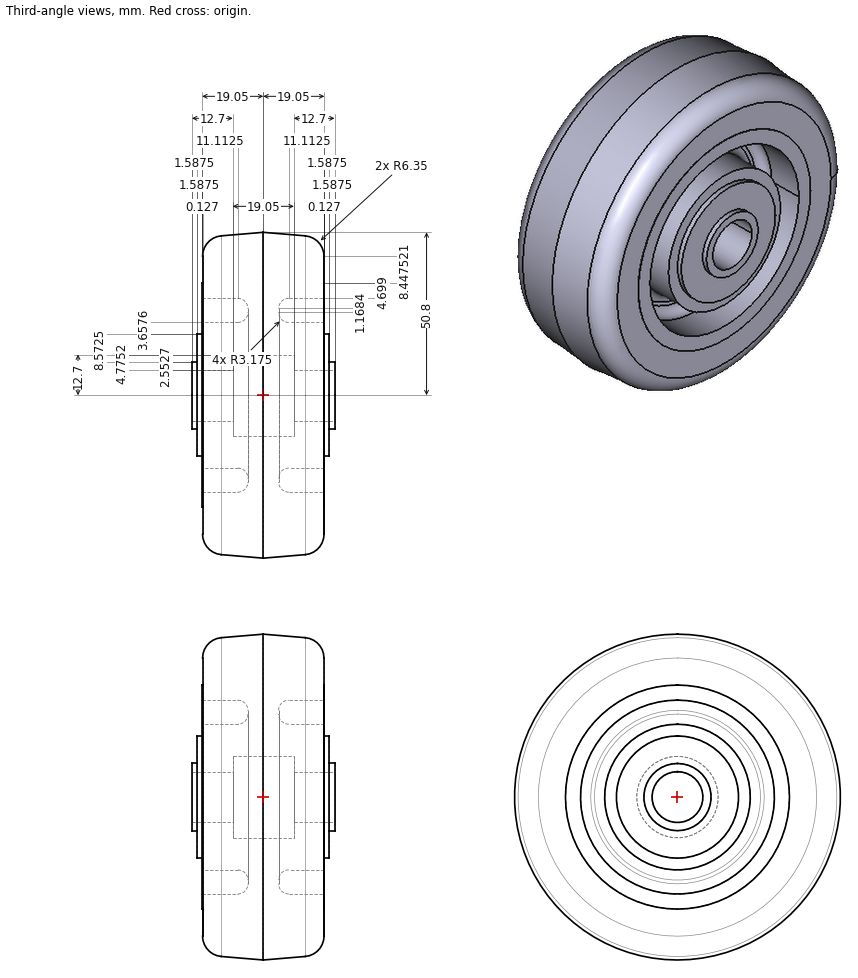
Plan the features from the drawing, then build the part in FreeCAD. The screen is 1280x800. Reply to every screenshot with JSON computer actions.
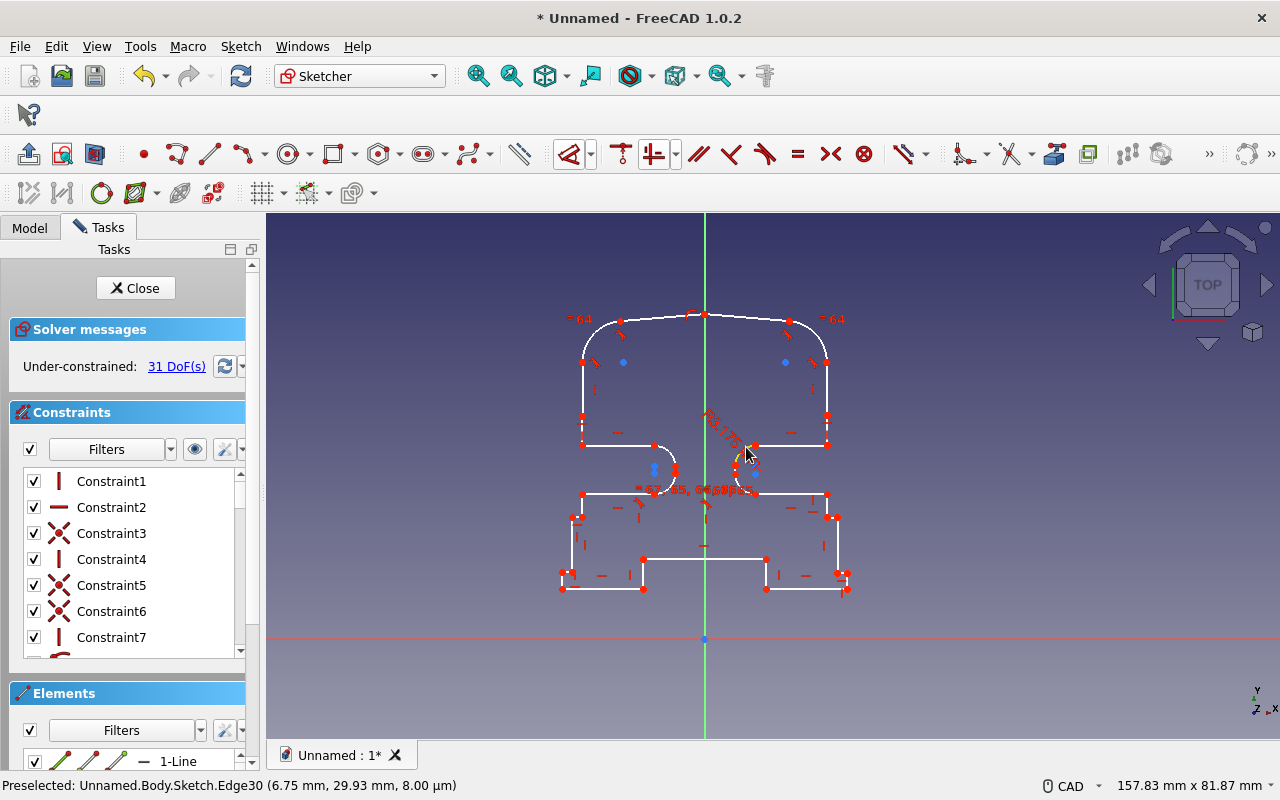
{"action": "left_click", "coordinate": [823, 344]}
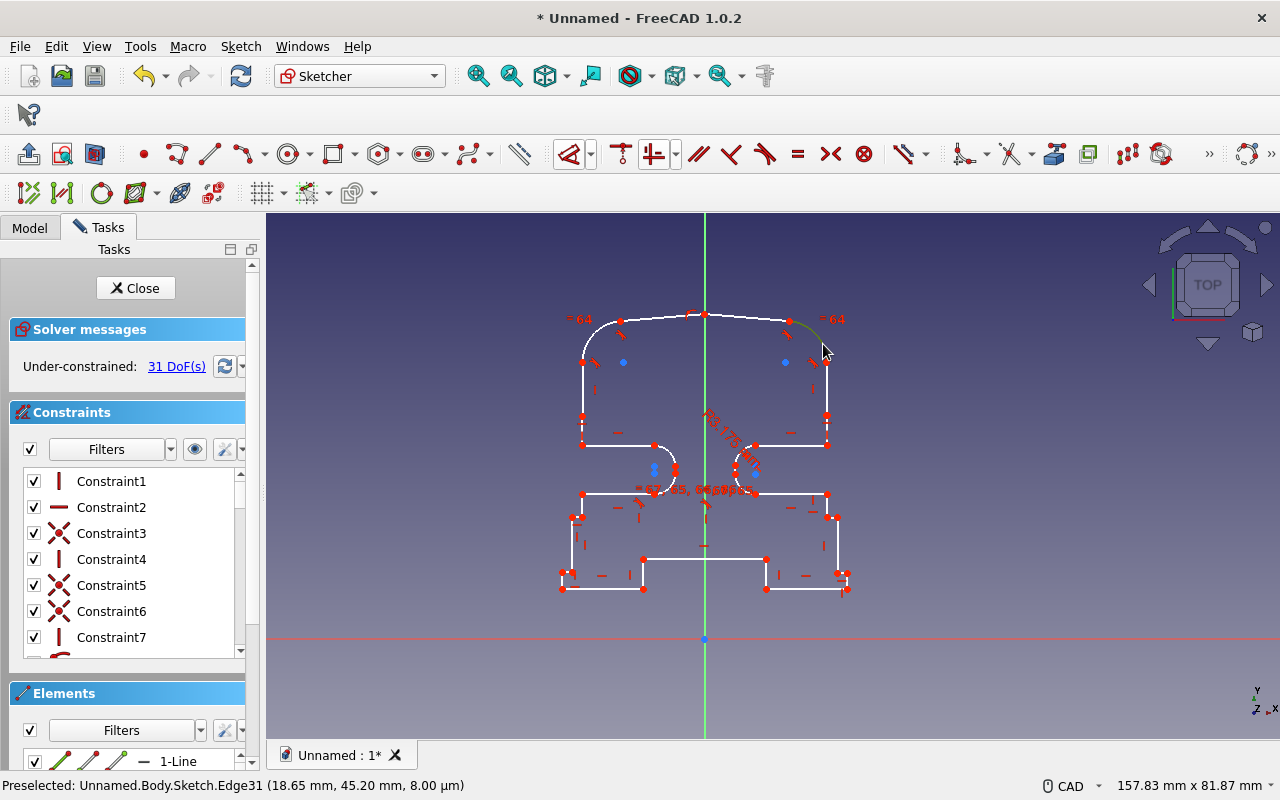
{"action": "left_click", "coordinate": [590, 154]}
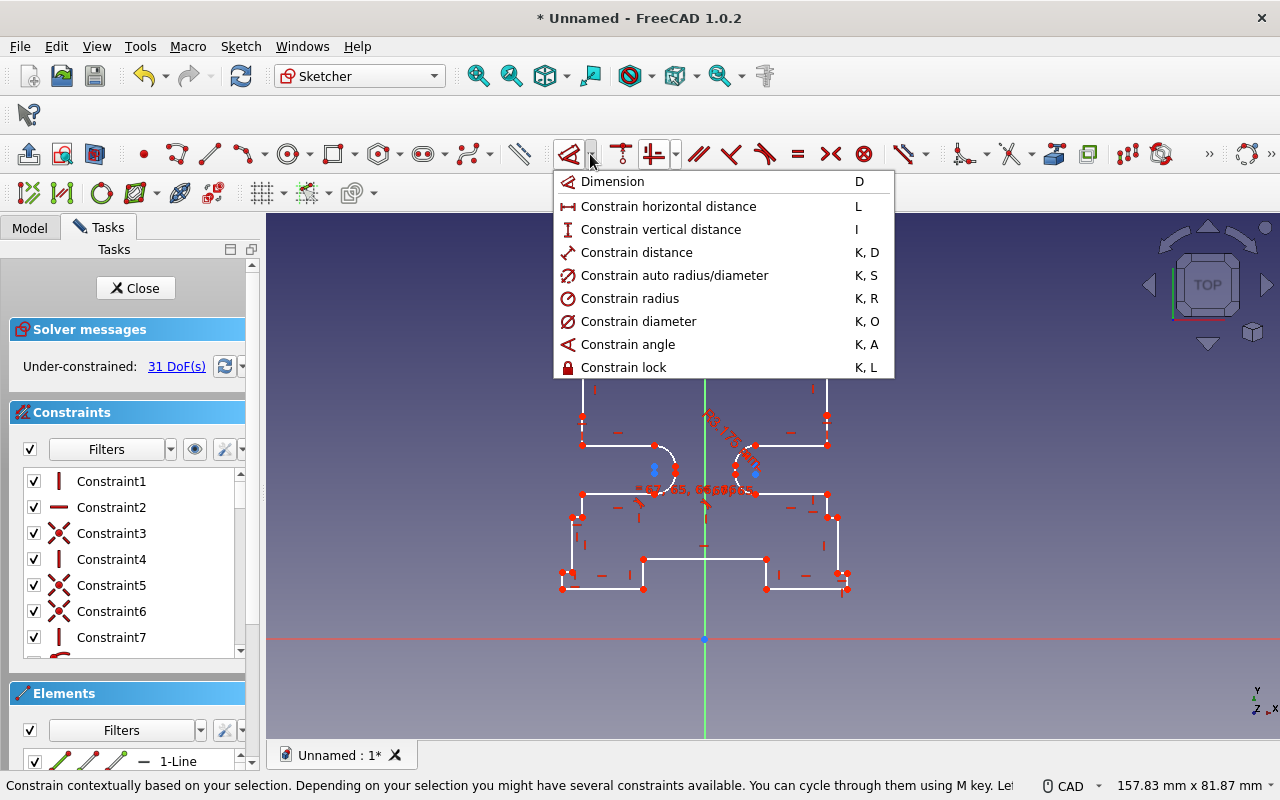
{"action": "left_click", "coordinate": [724, 298]}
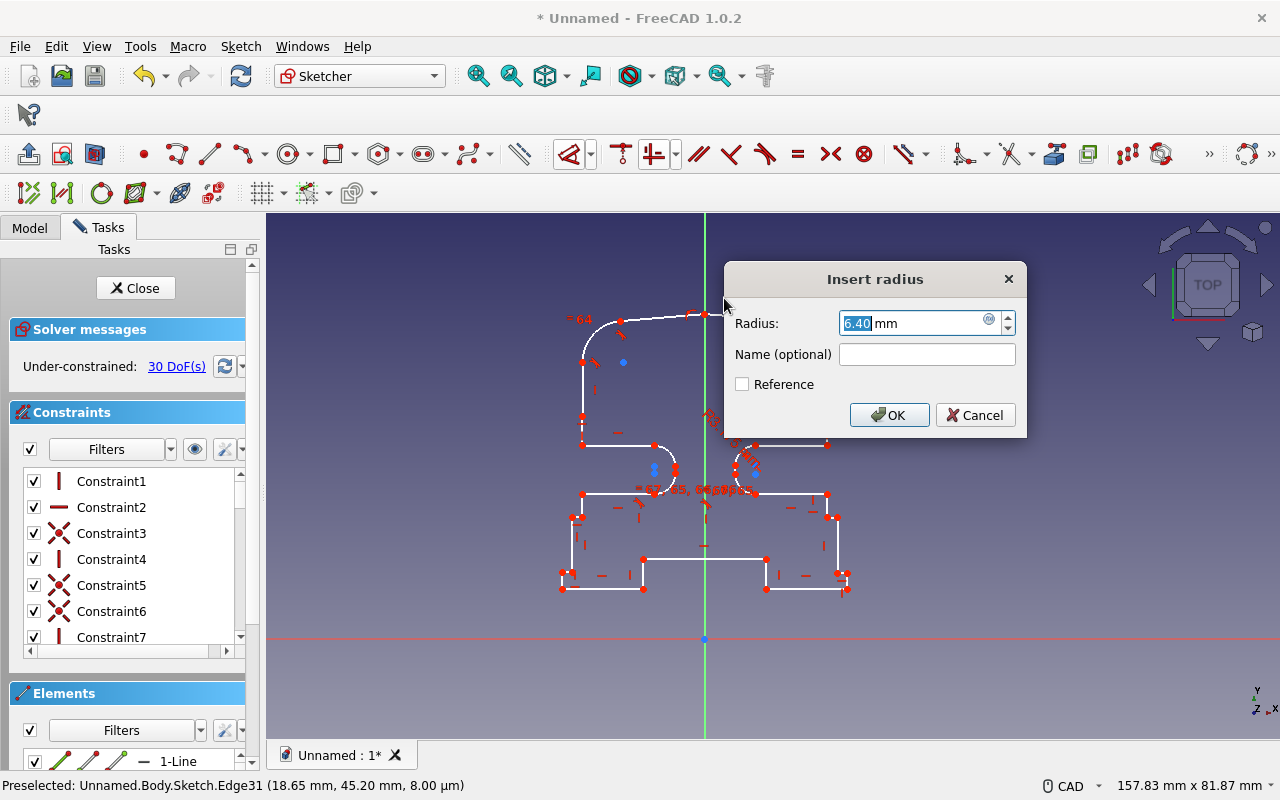
{"action": "type", "text": "6.35"}
{"action": "key", "text": "Return"}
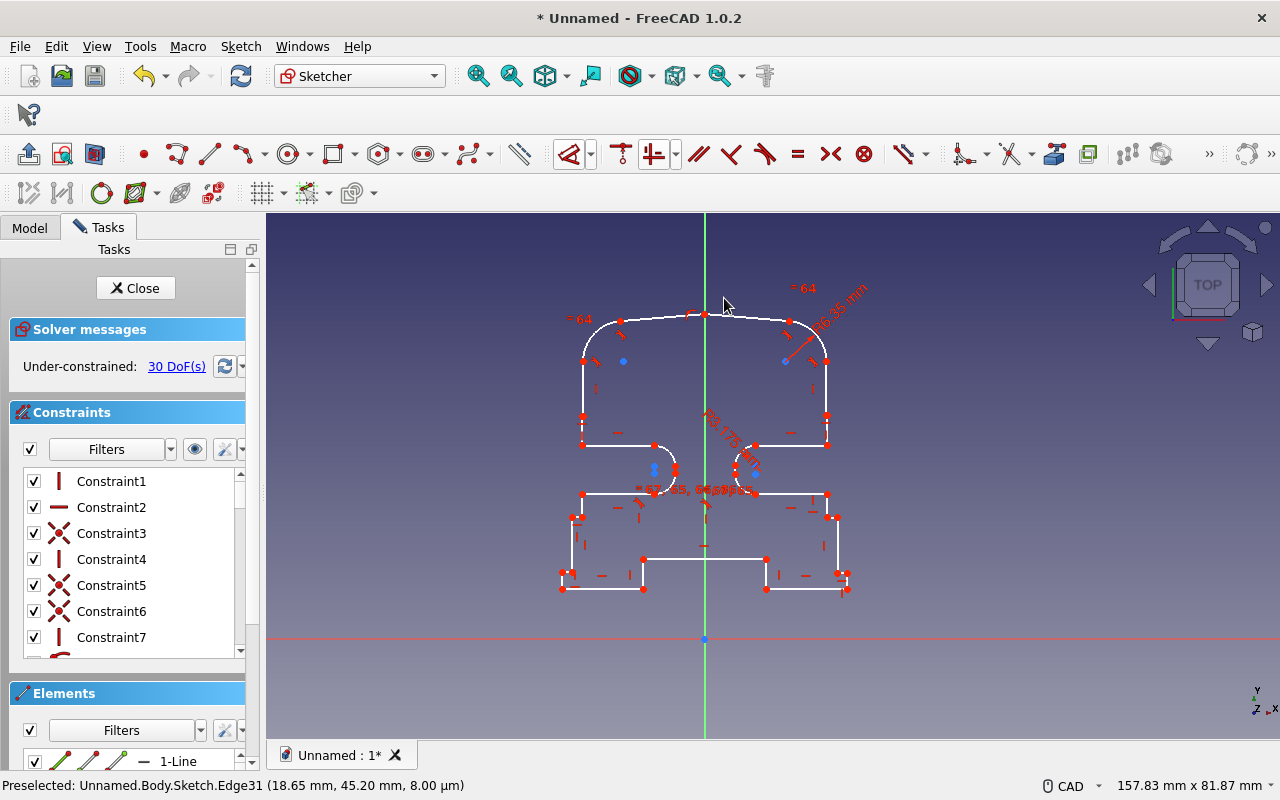
{"action": "left_click", "coordinate": [587, 589]}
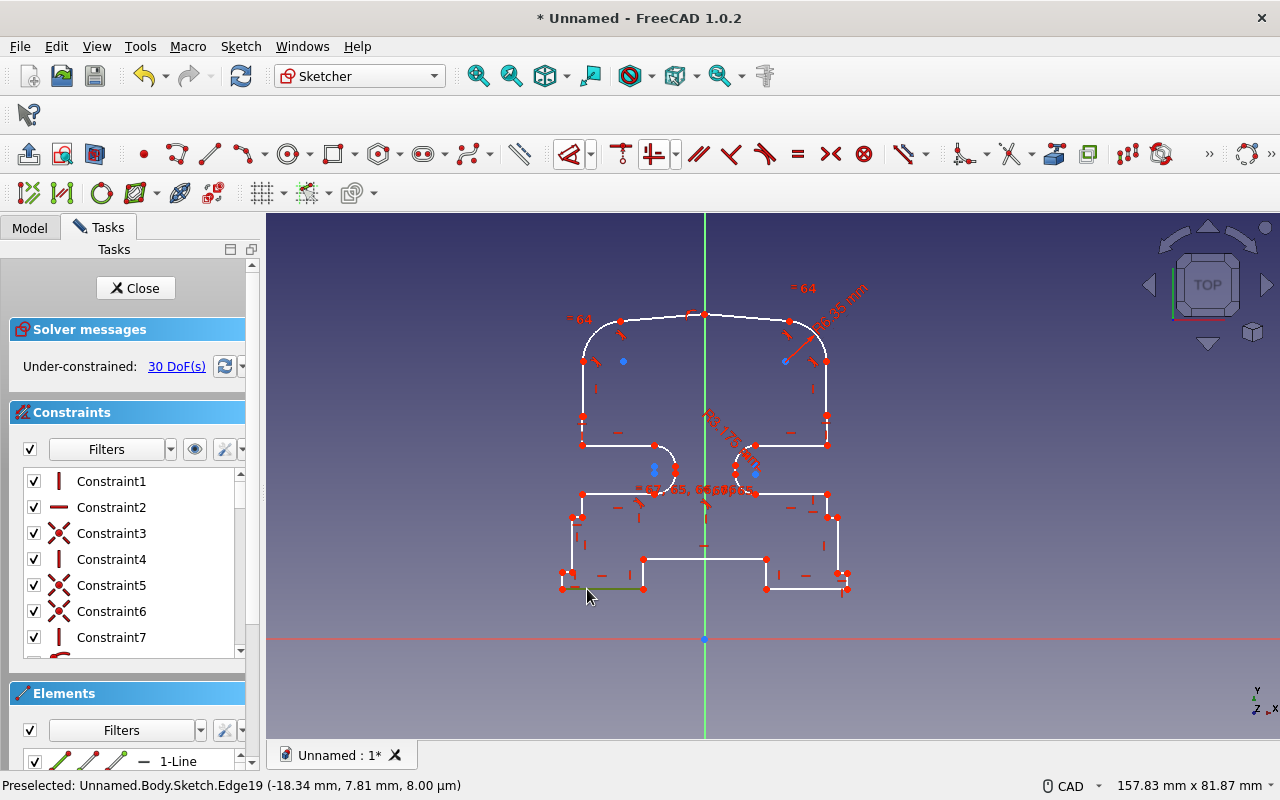
{"action": "left_click", "coordinate": [590, 154]}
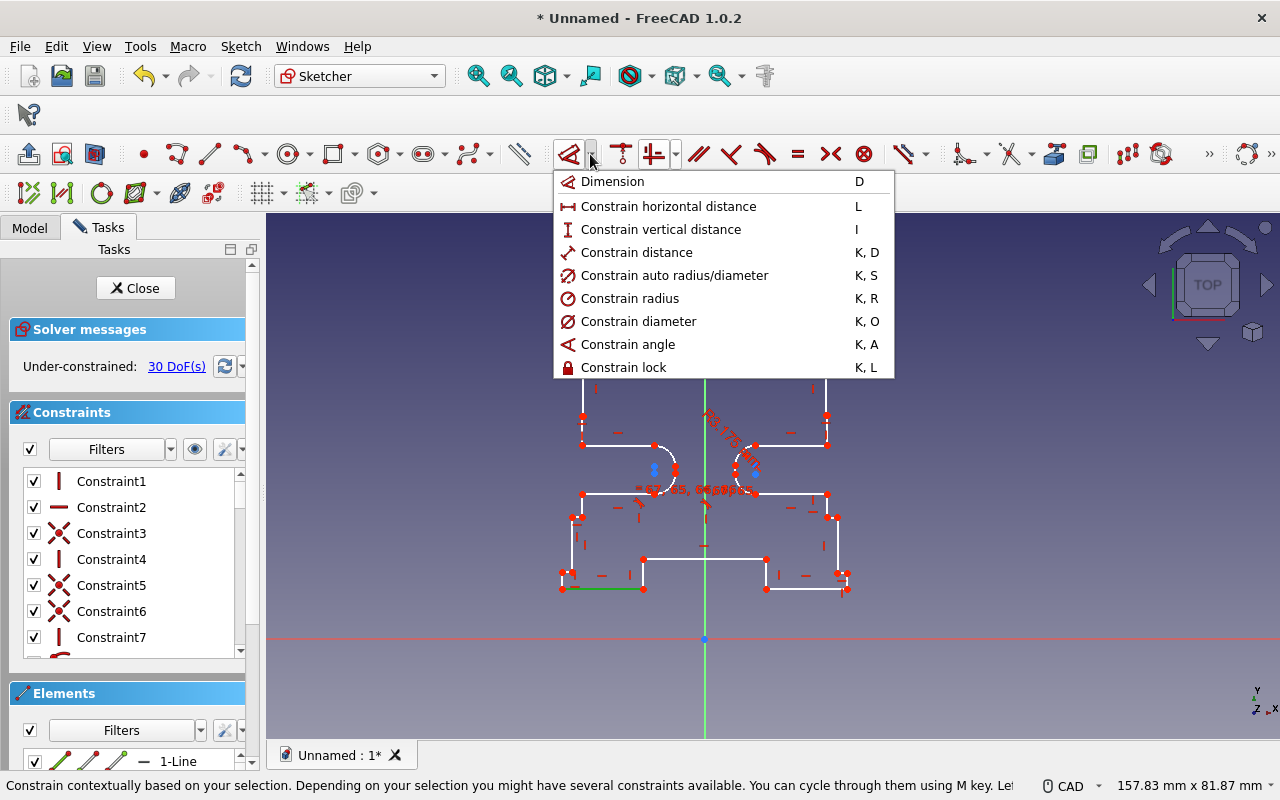
{"action": "left_click", "coordinate": [724, 206]}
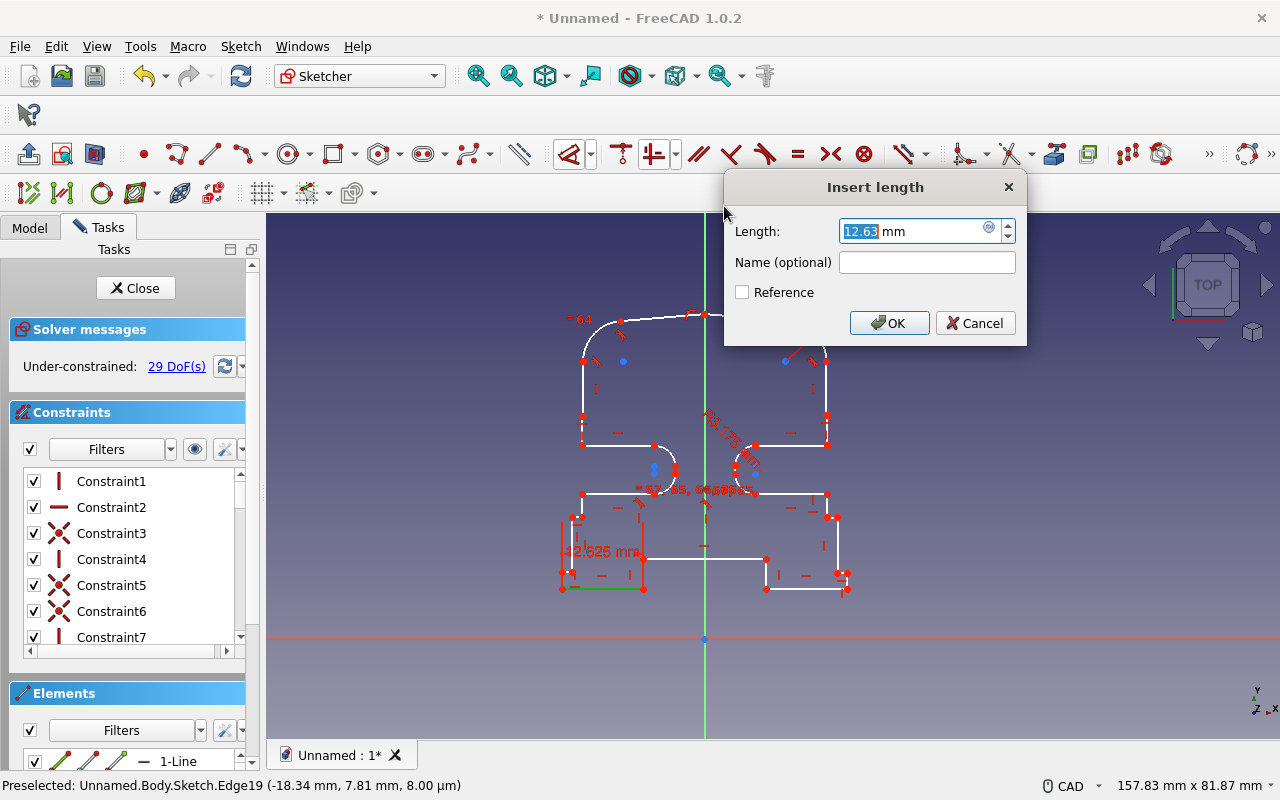
{"action": "type", "text": "12.7"}
{"action": "key", "text": "Return"}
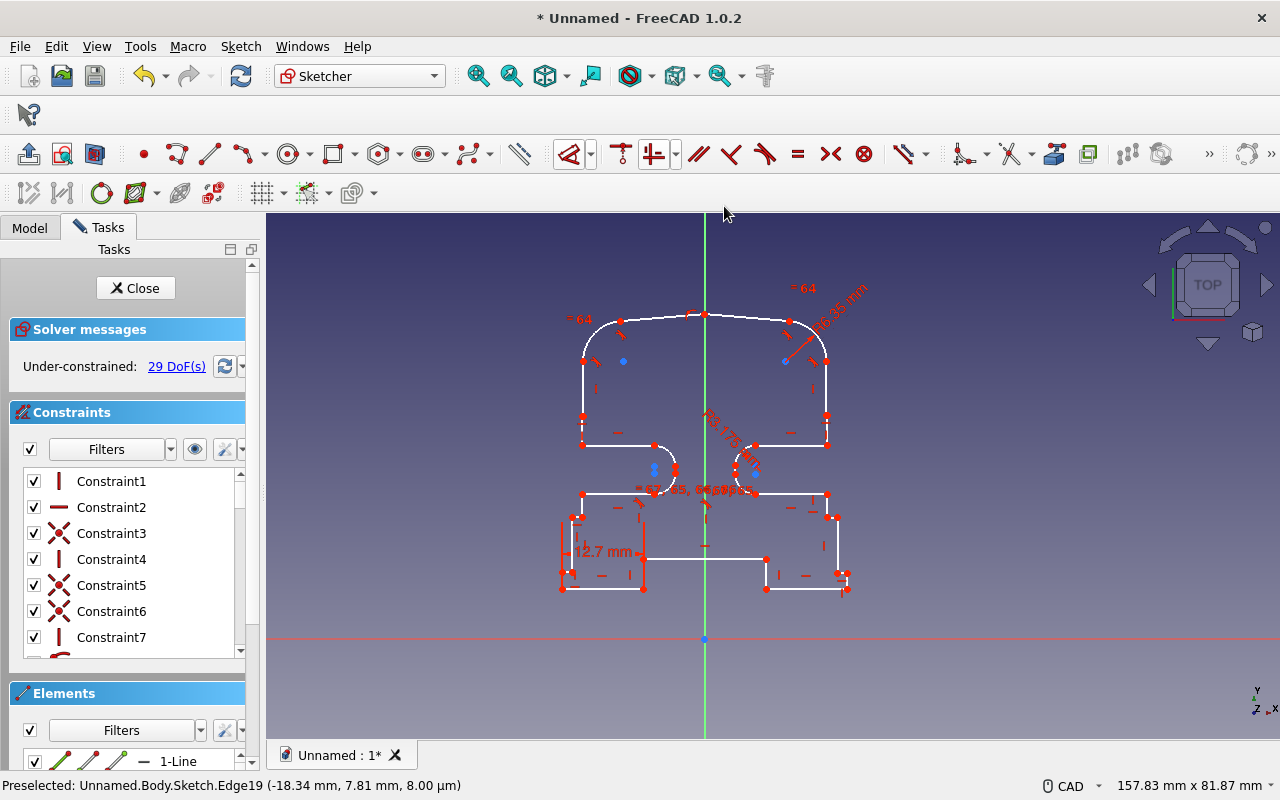
{"action": "left_click", "coordinate": [791, 589]}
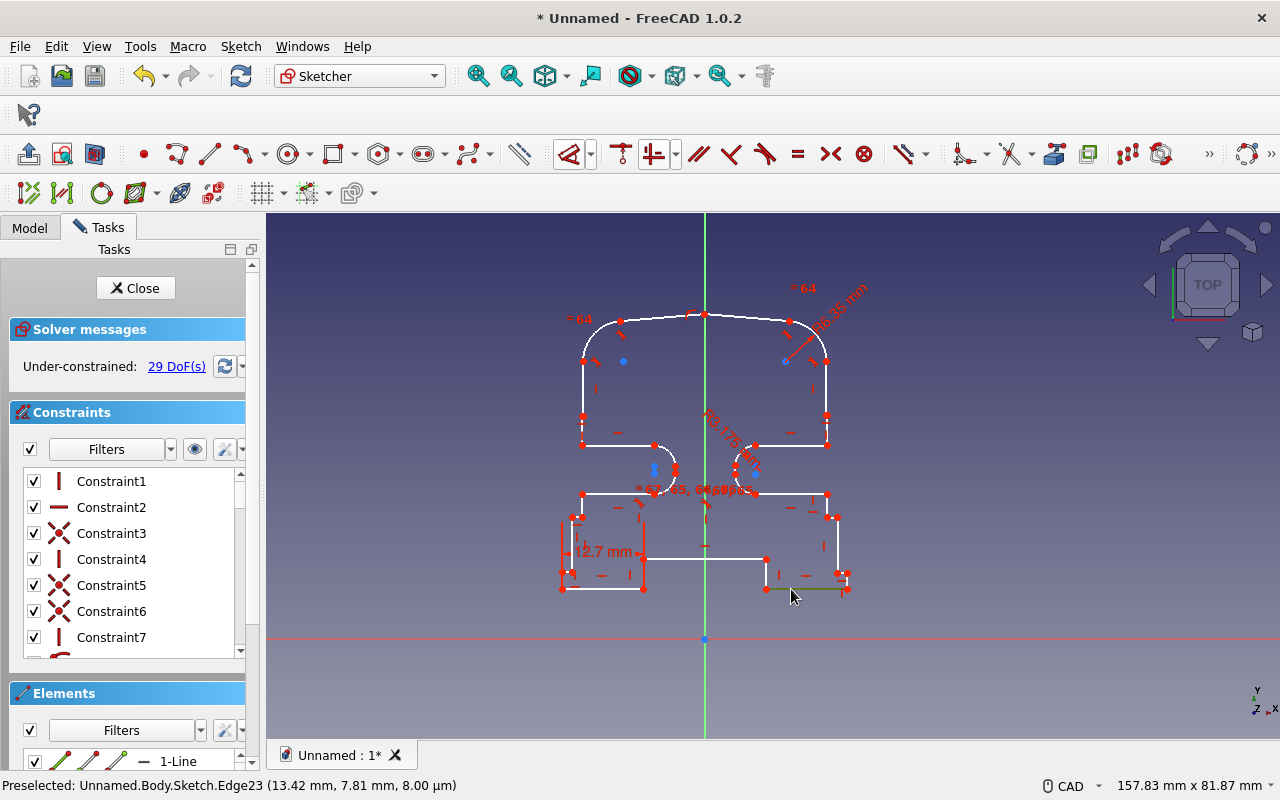
{"action": "key", "text": "l"}